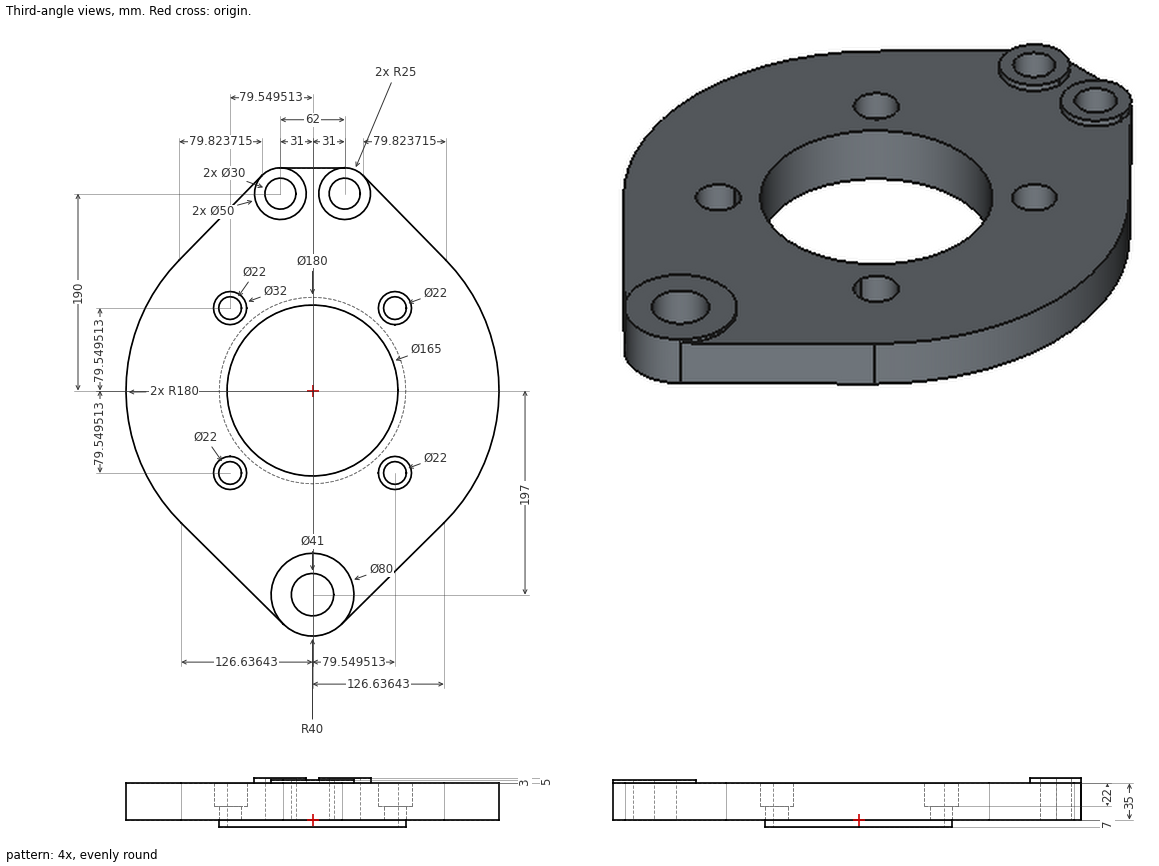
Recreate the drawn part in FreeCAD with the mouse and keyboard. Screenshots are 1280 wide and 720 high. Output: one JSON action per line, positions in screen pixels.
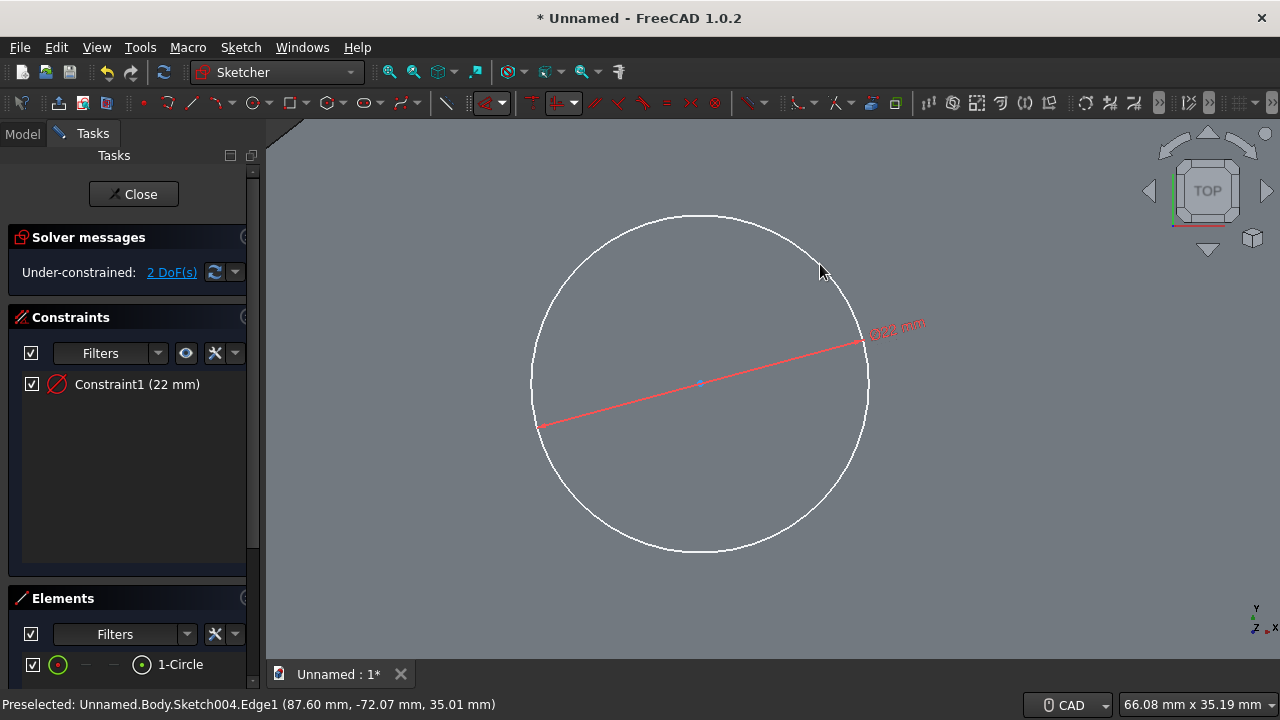
{"action": "left_click", "coordinate": [700, 384]}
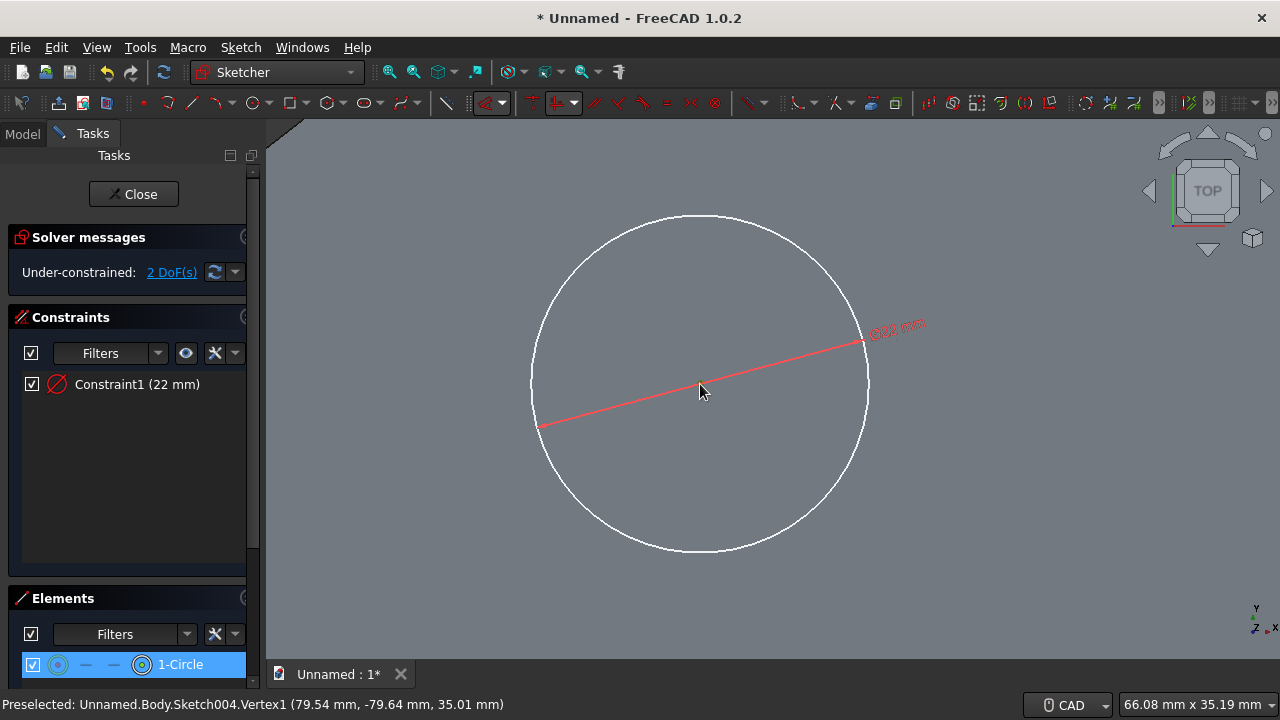
{"action": "left_click", "coordinate": [504, 104]}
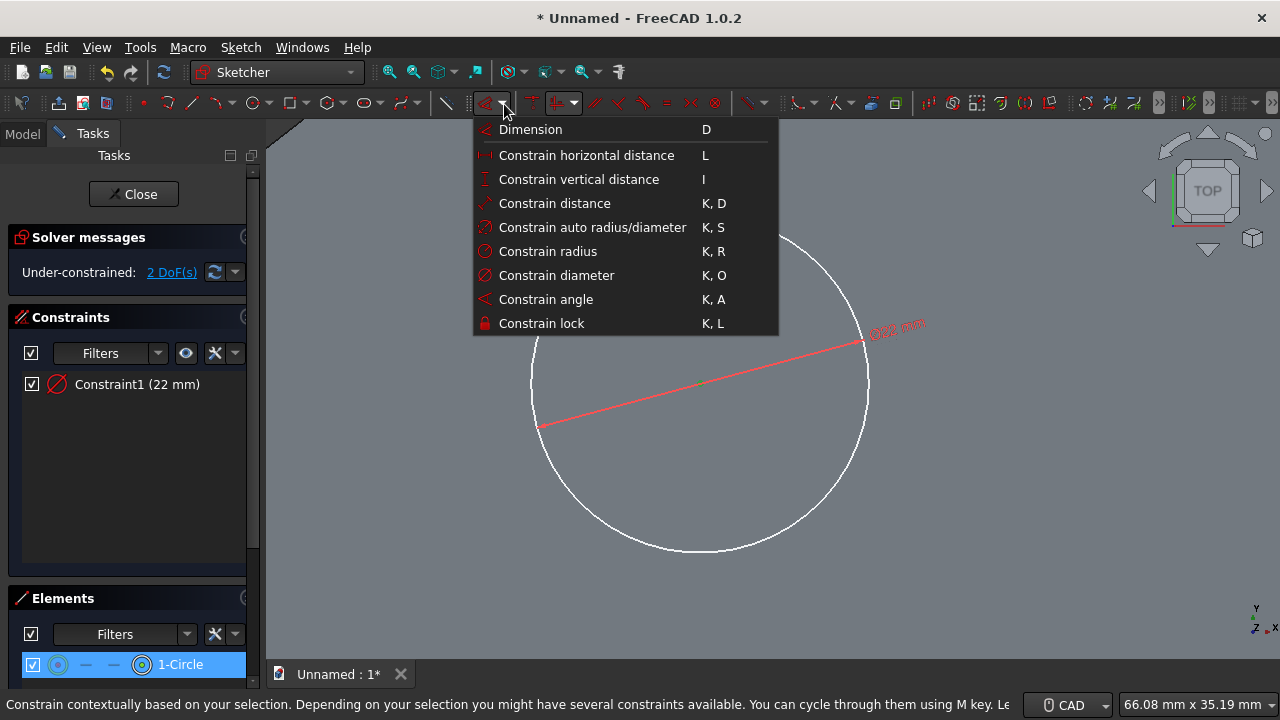
{"action": "left_click", "coordinate": [626, 155]}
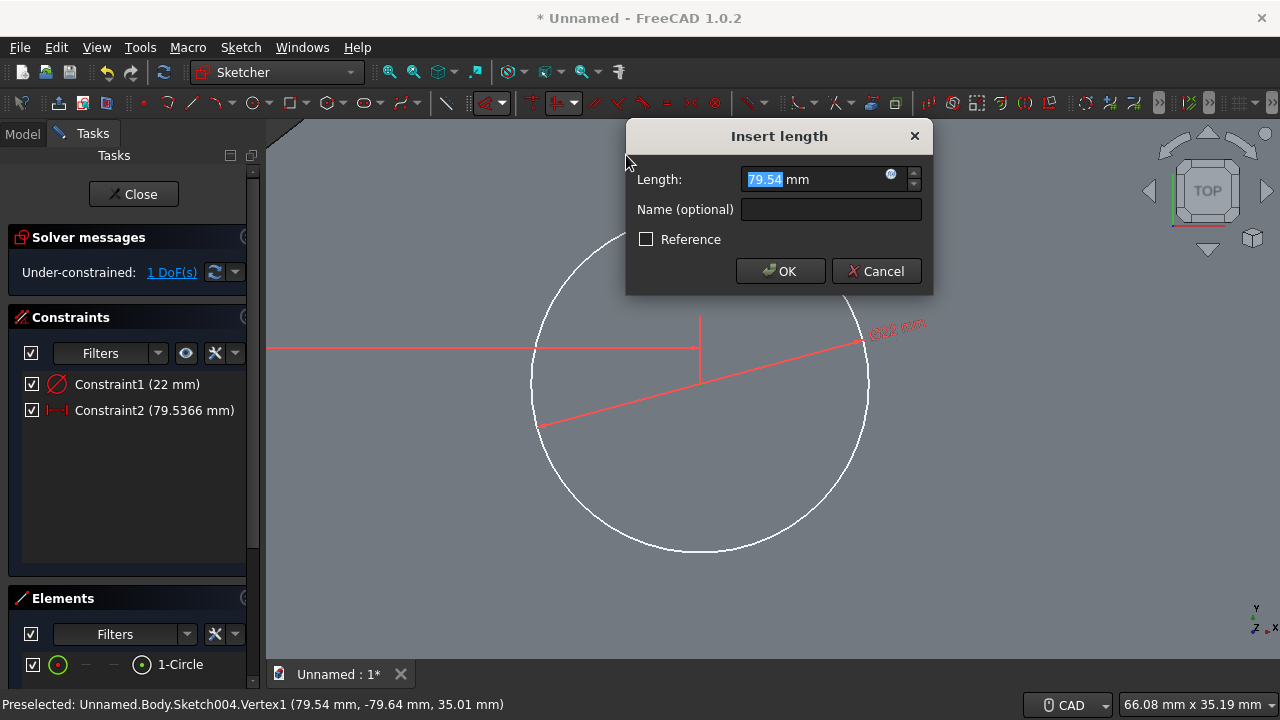
{"action": "type", "text": "79.549513"}
{"action": "key", "text": "Return"}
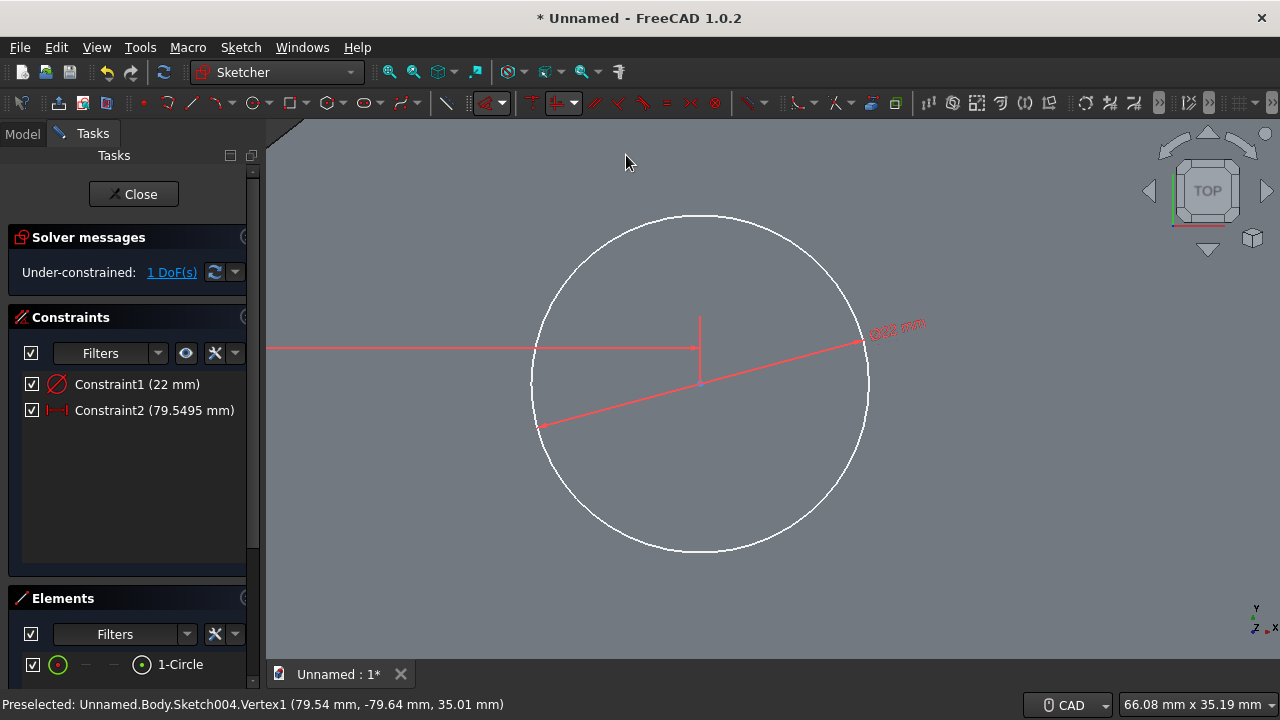
{"action": "left_click", "coordinate": [700, 384]}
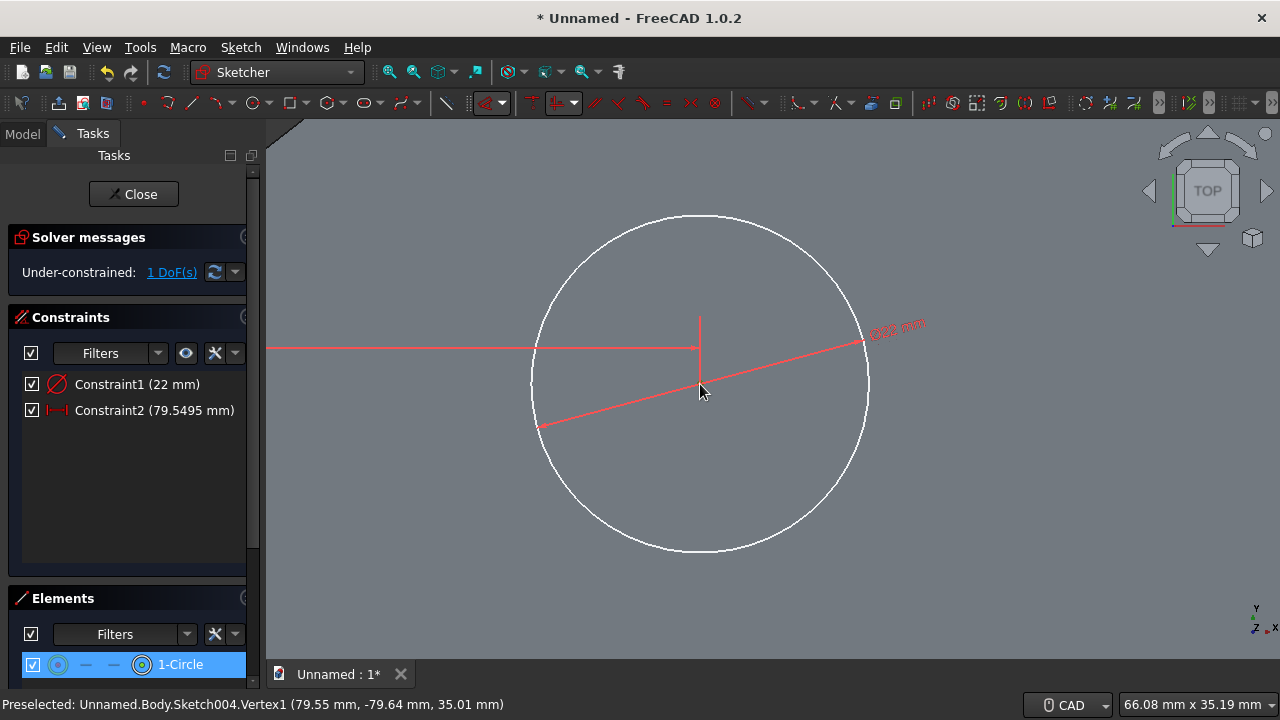
{"action": "left_click", "coordinate": [504, 104]}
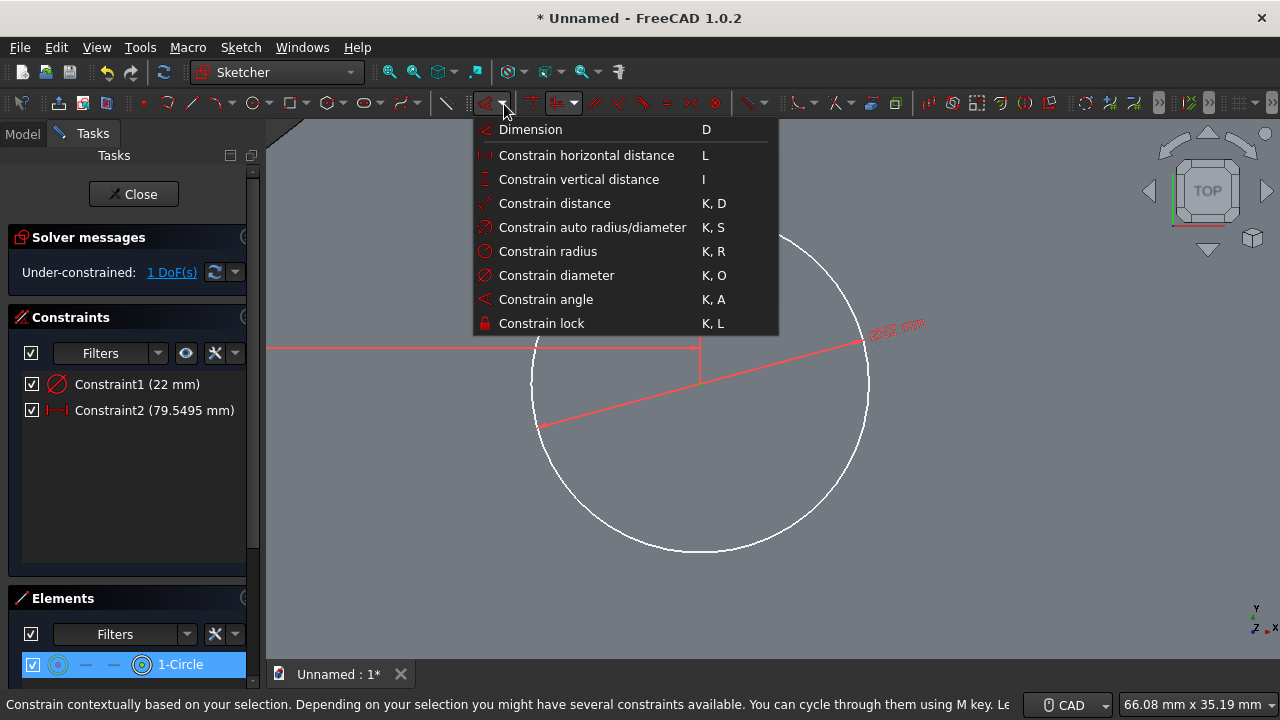
{"action": "left_click", "coordinate": [626, 179]}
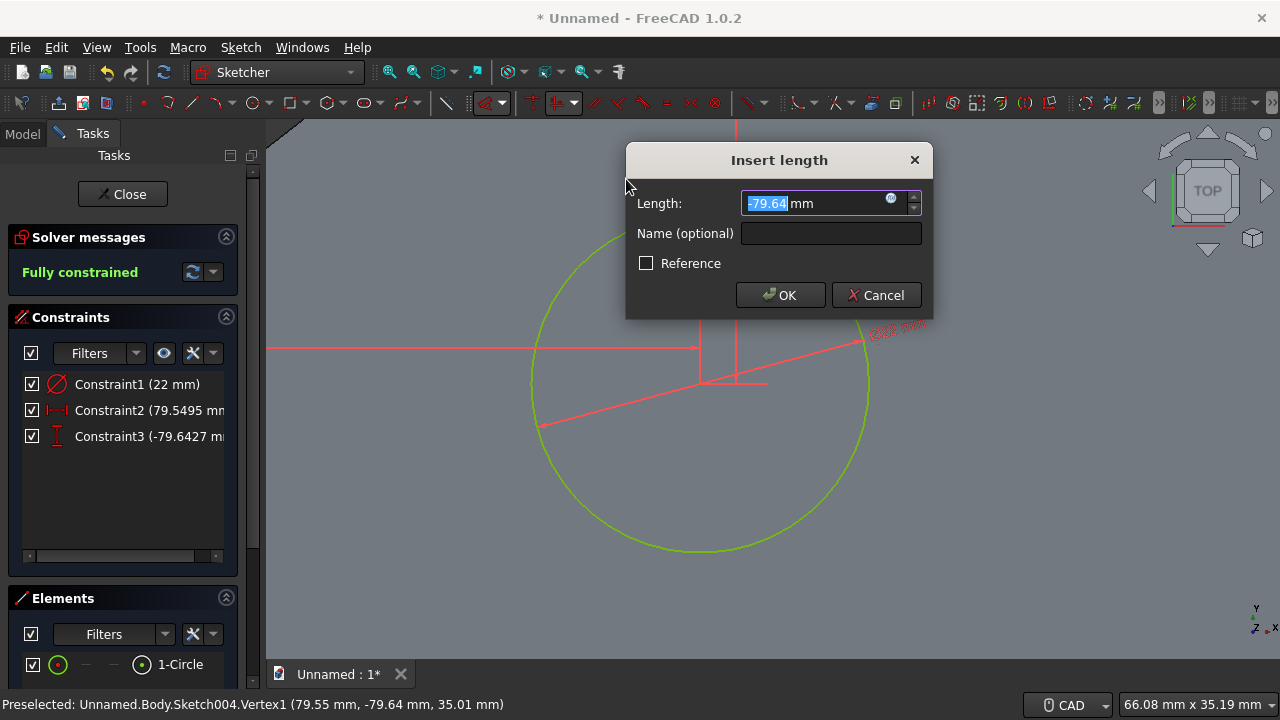
{"action": "type", "text": "-79.549513"}
{"action": "key", "text": "Return"}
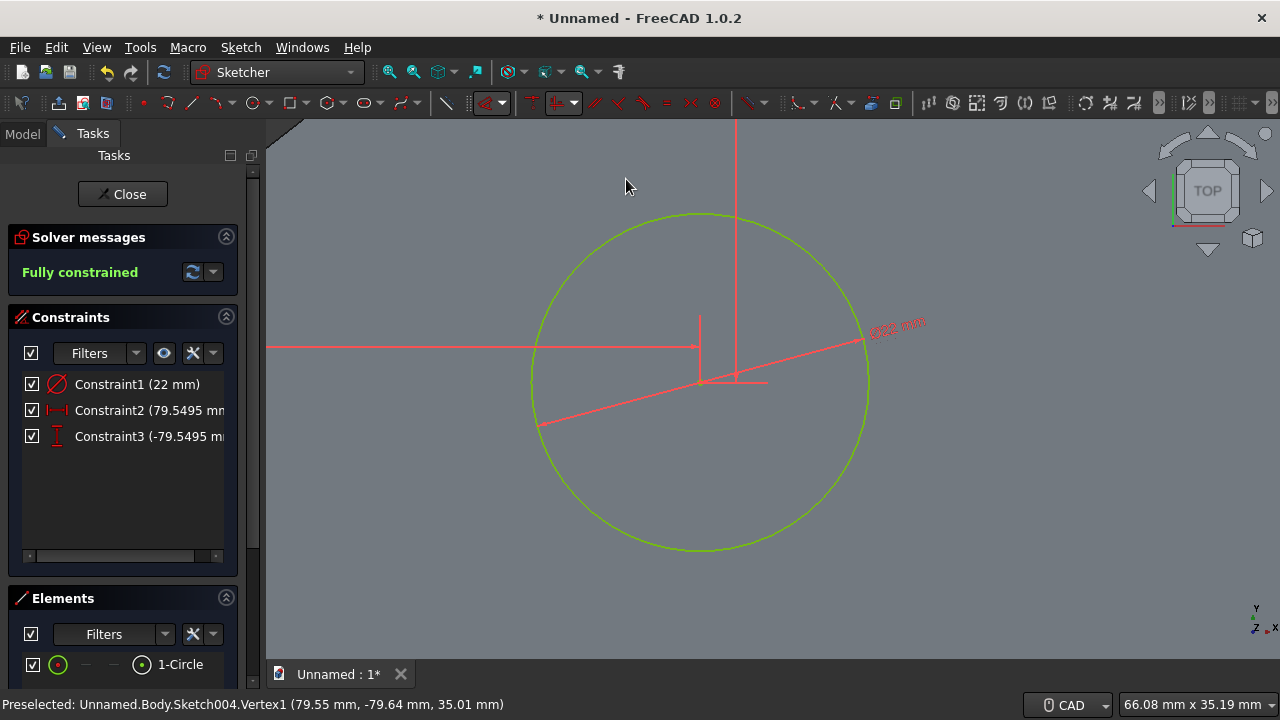
{"action": "left_click", "coordinate": [123, 194]}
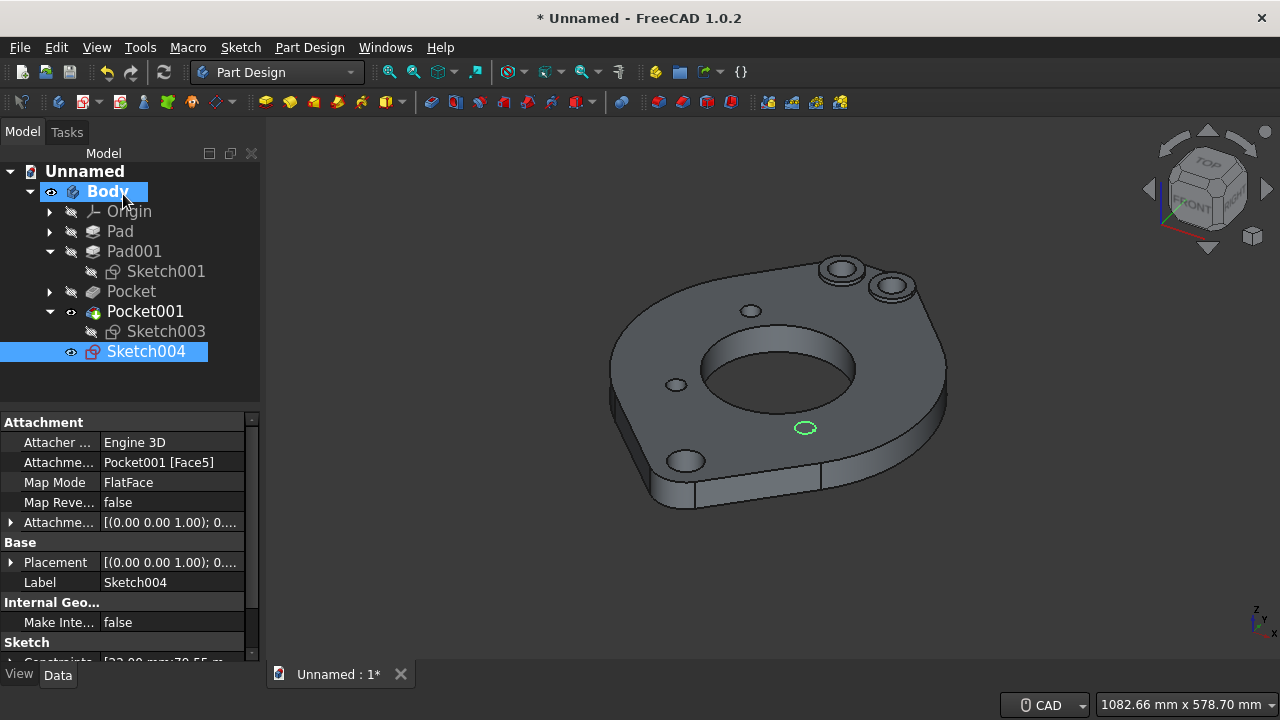
{"action": "left_click", "coordinate": [432, 102]}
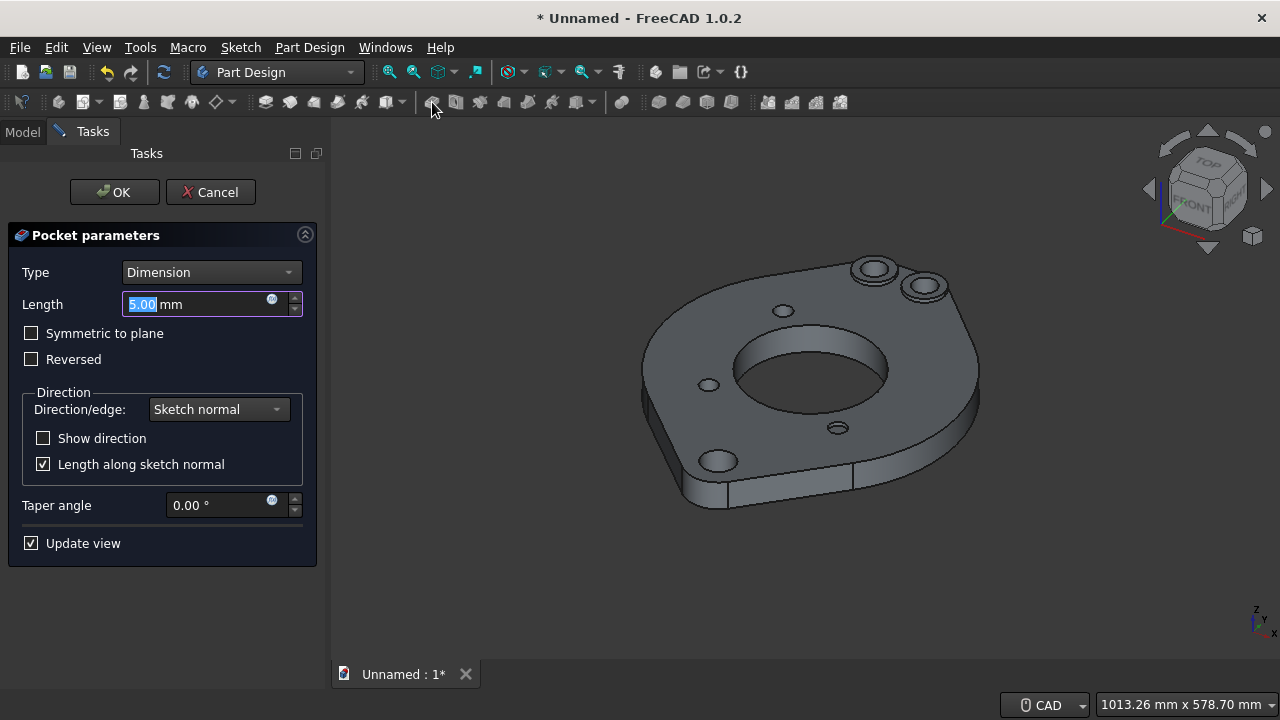
{"action": "left_click", "coordinate": [212, 272]}